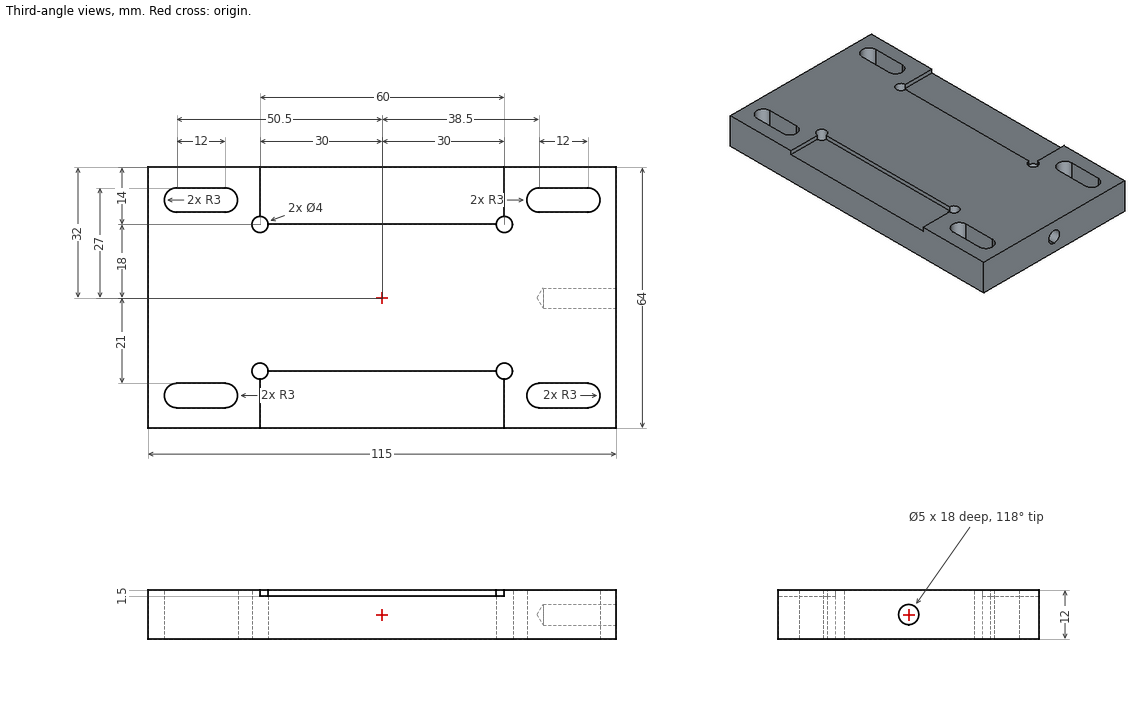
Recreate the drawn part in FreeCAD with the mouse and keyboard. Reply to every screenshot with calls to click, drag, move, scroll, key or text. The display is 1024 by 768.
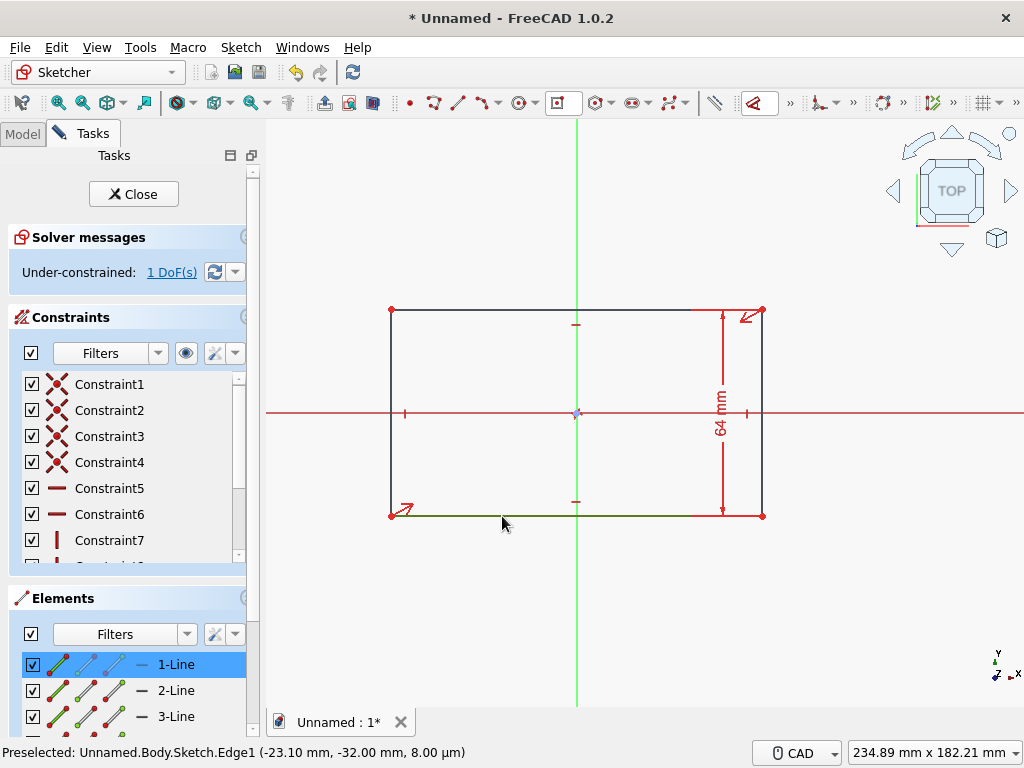
click(772, 104)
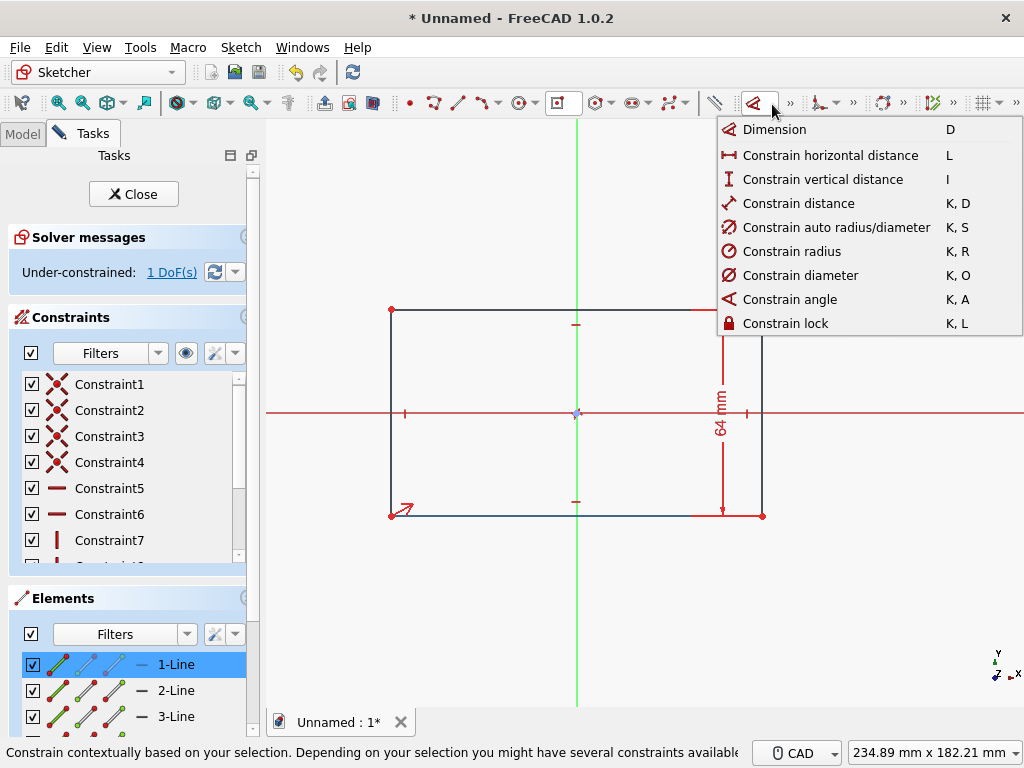
click(870, 155)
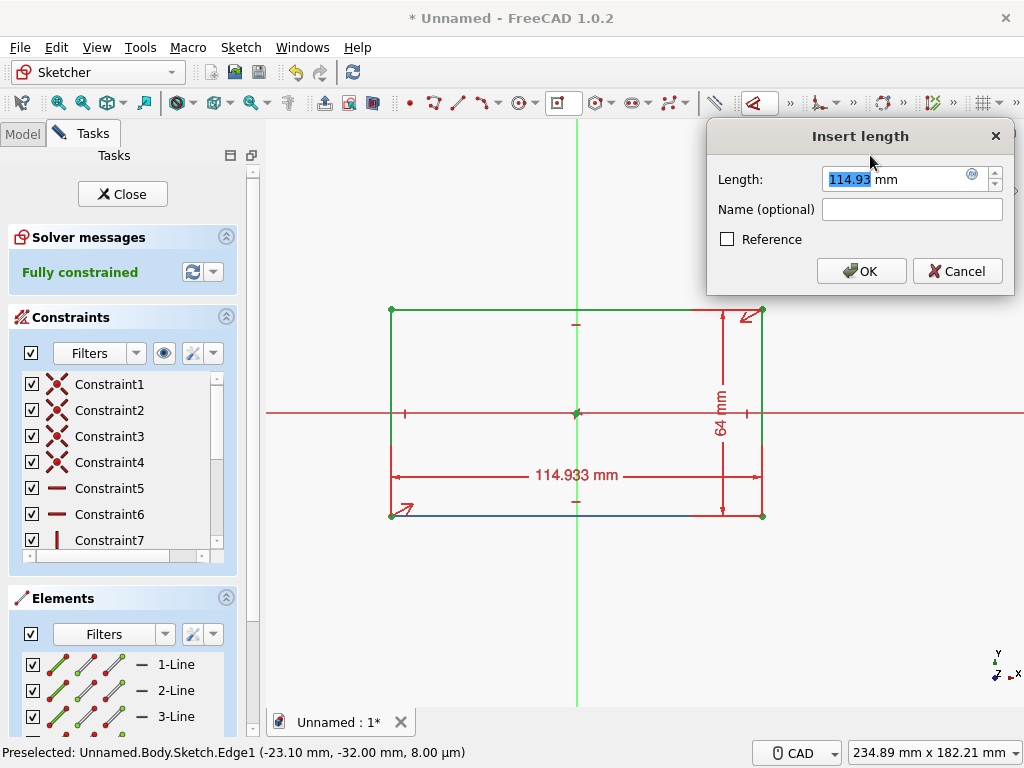
text(115)
key(Return)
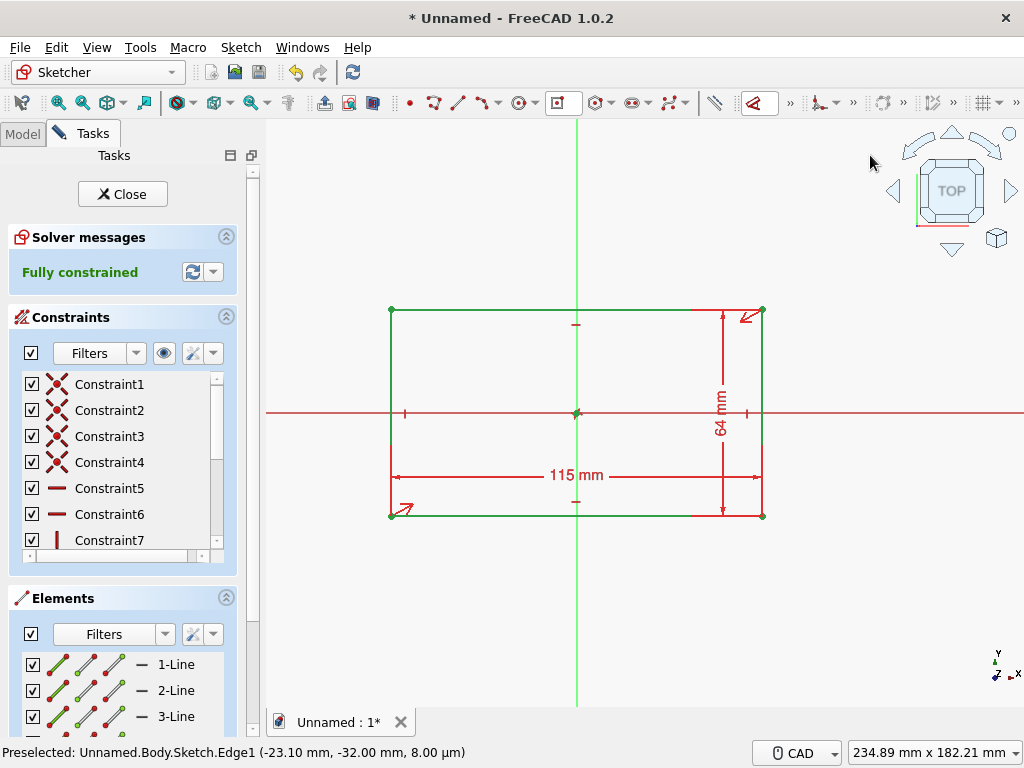
click(123, 194)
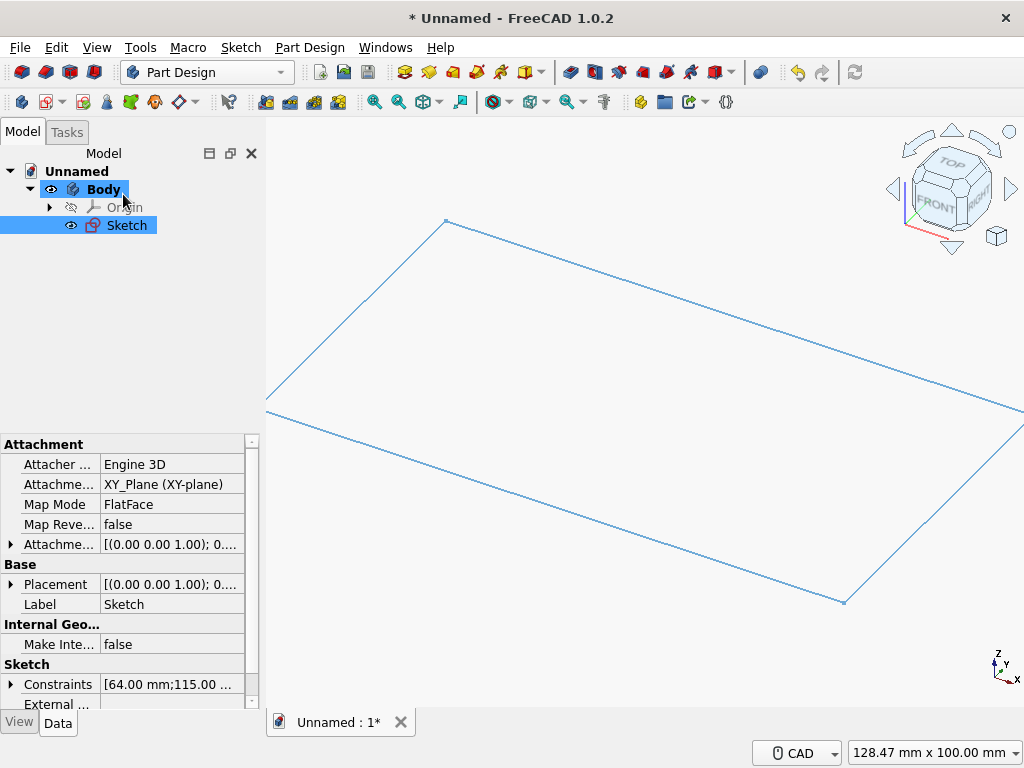
click(406, 72)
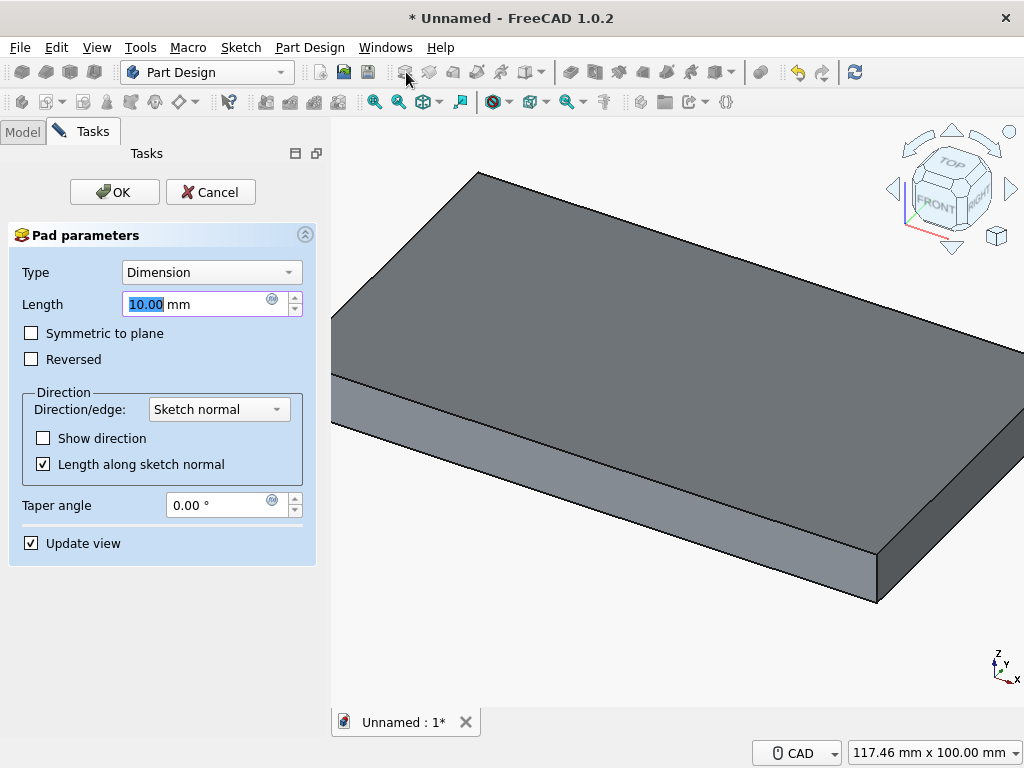
text(12)
key(Tab)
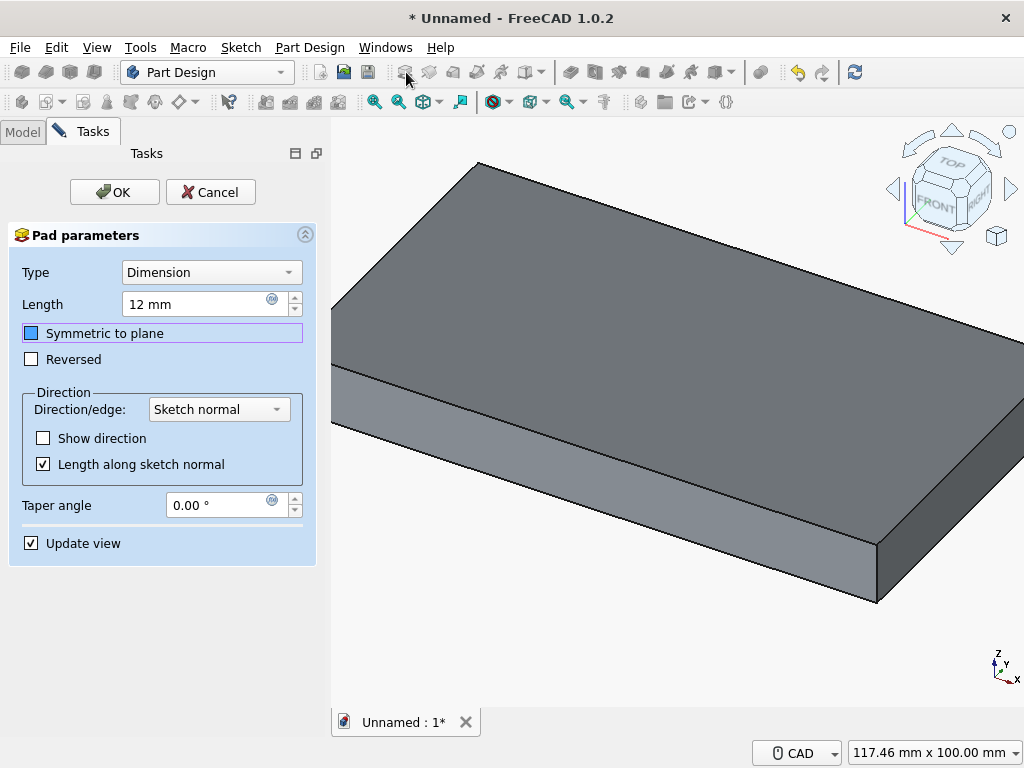
click(30, 333)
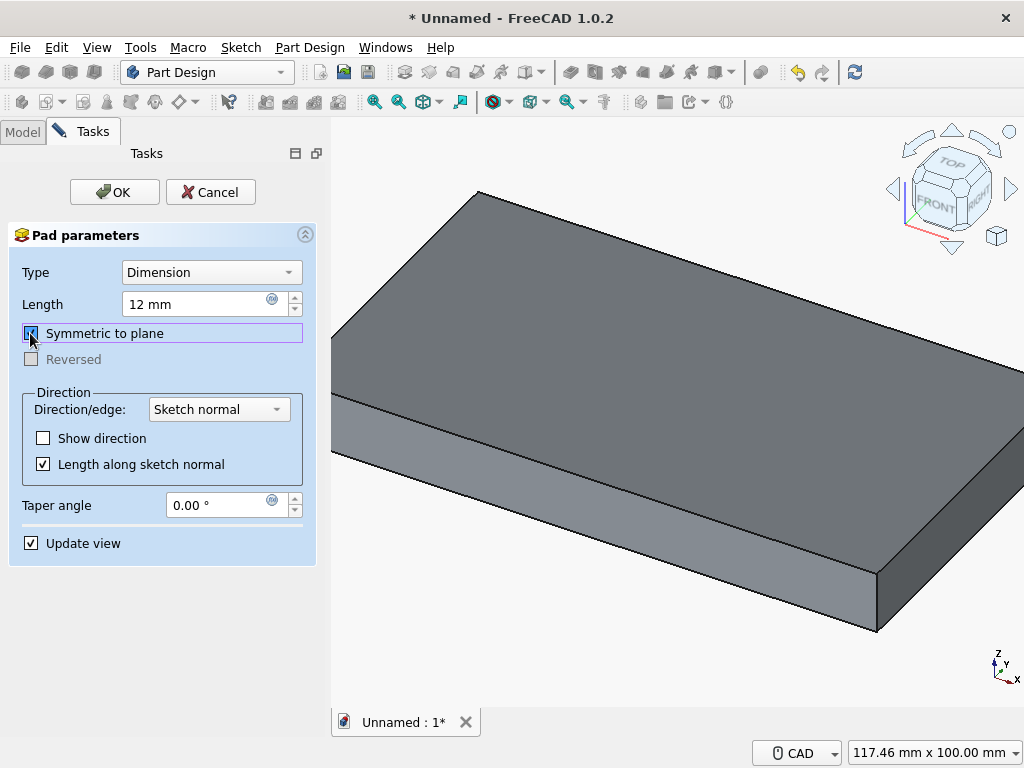
click(115, 192)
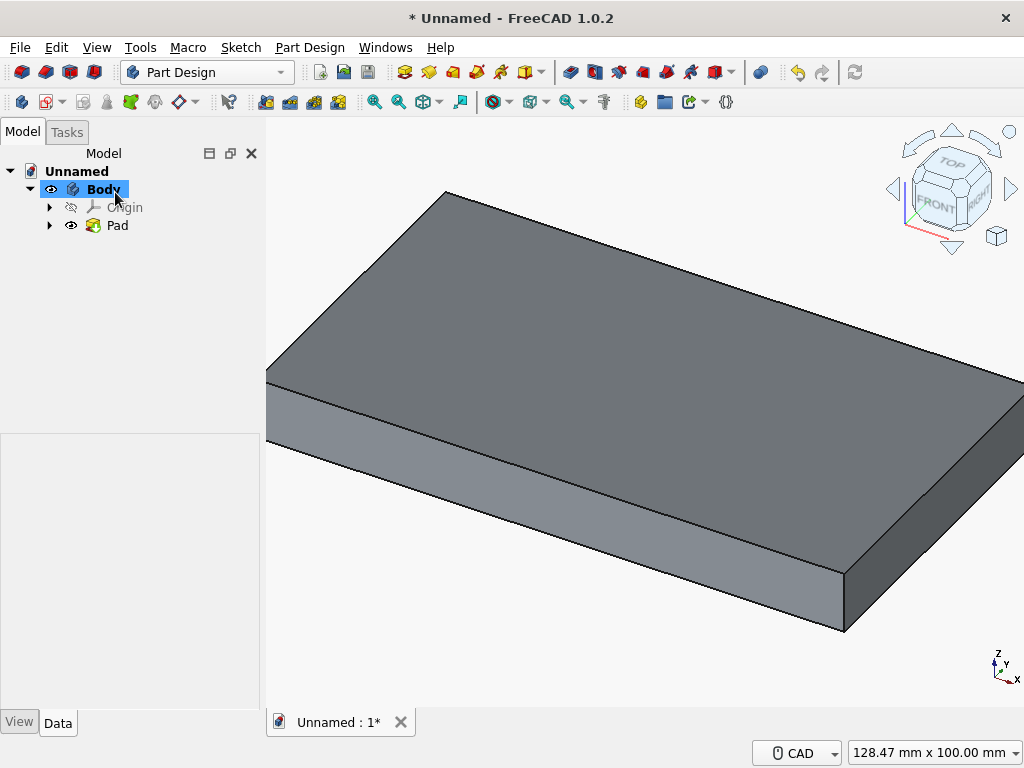
click(376, 102)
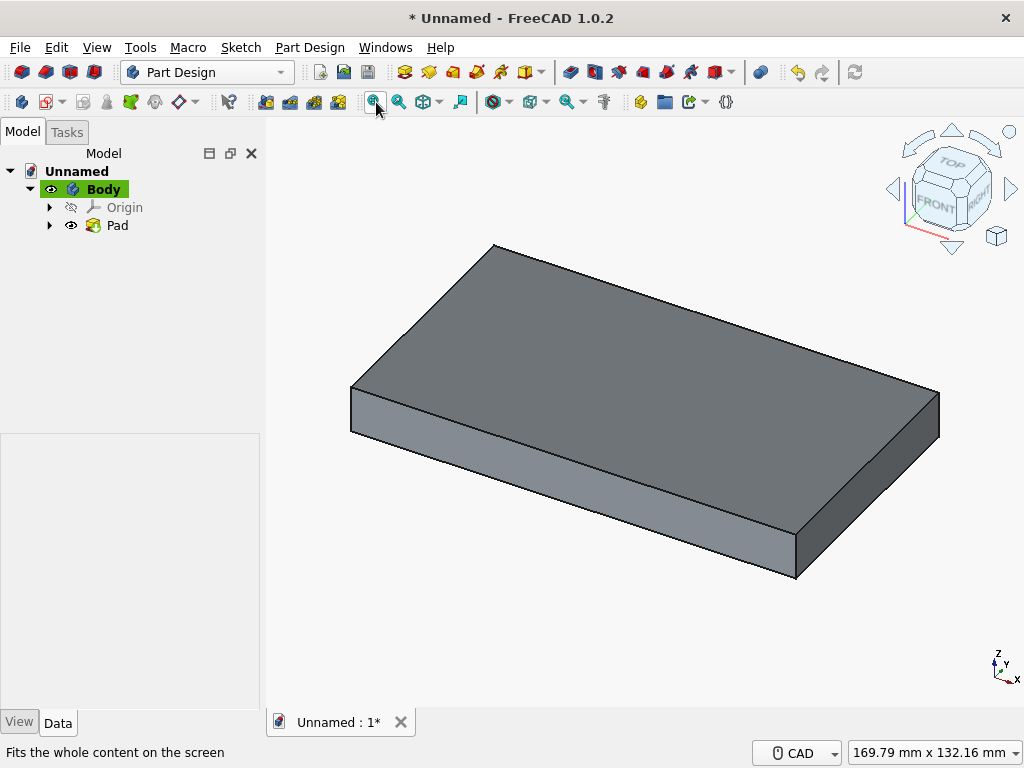
click(709, 410)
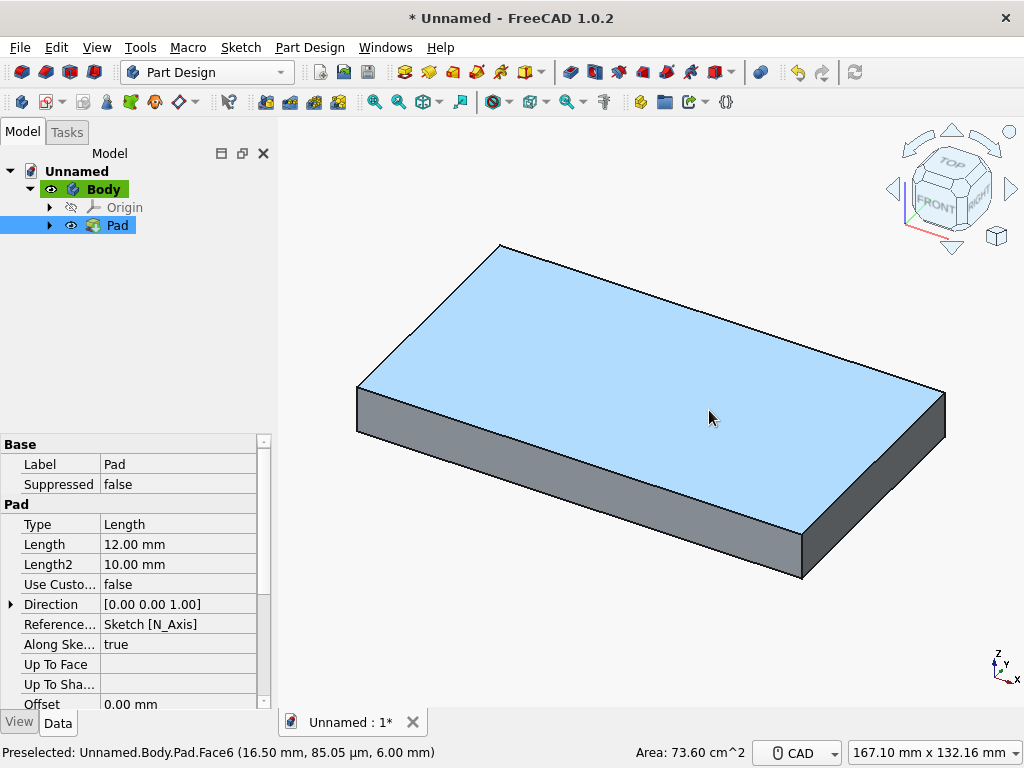
click(46, 102)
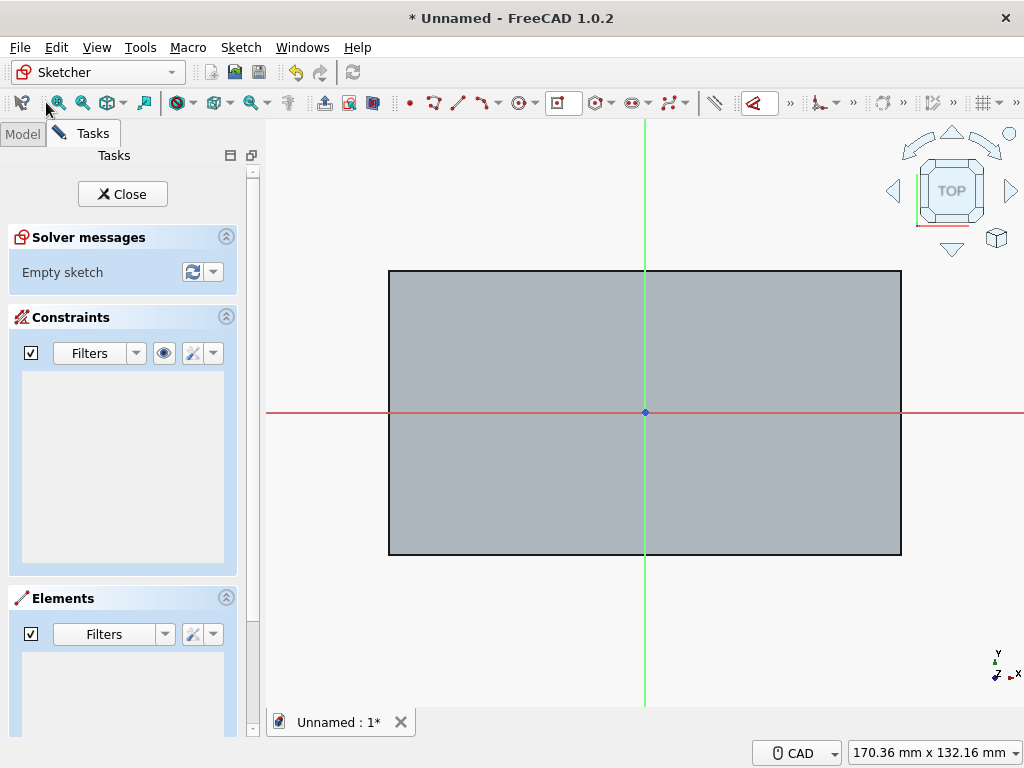
scroll(784, 197, up, 2)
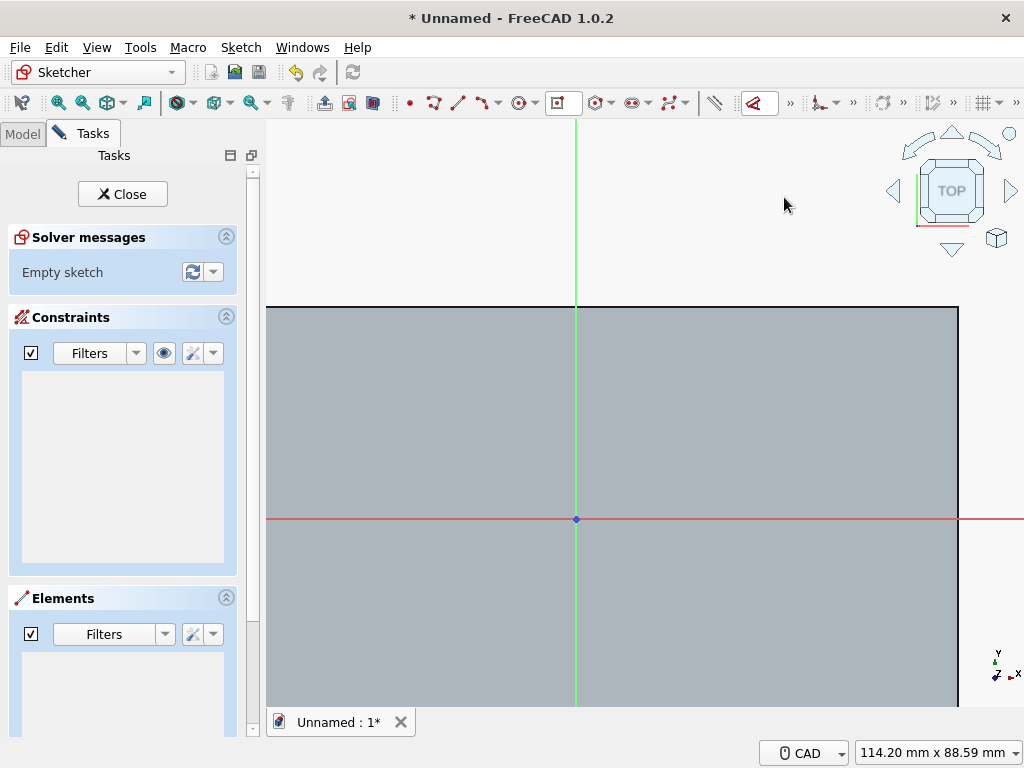
key(g)
key(r)